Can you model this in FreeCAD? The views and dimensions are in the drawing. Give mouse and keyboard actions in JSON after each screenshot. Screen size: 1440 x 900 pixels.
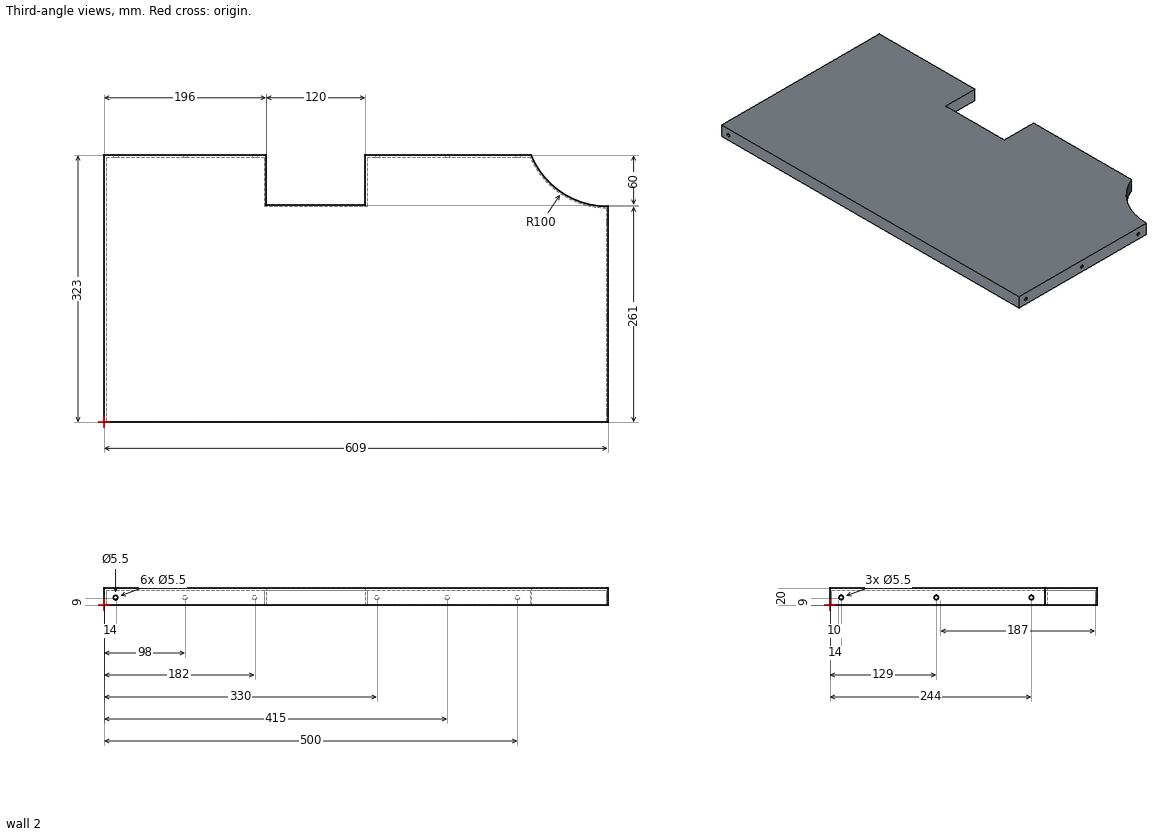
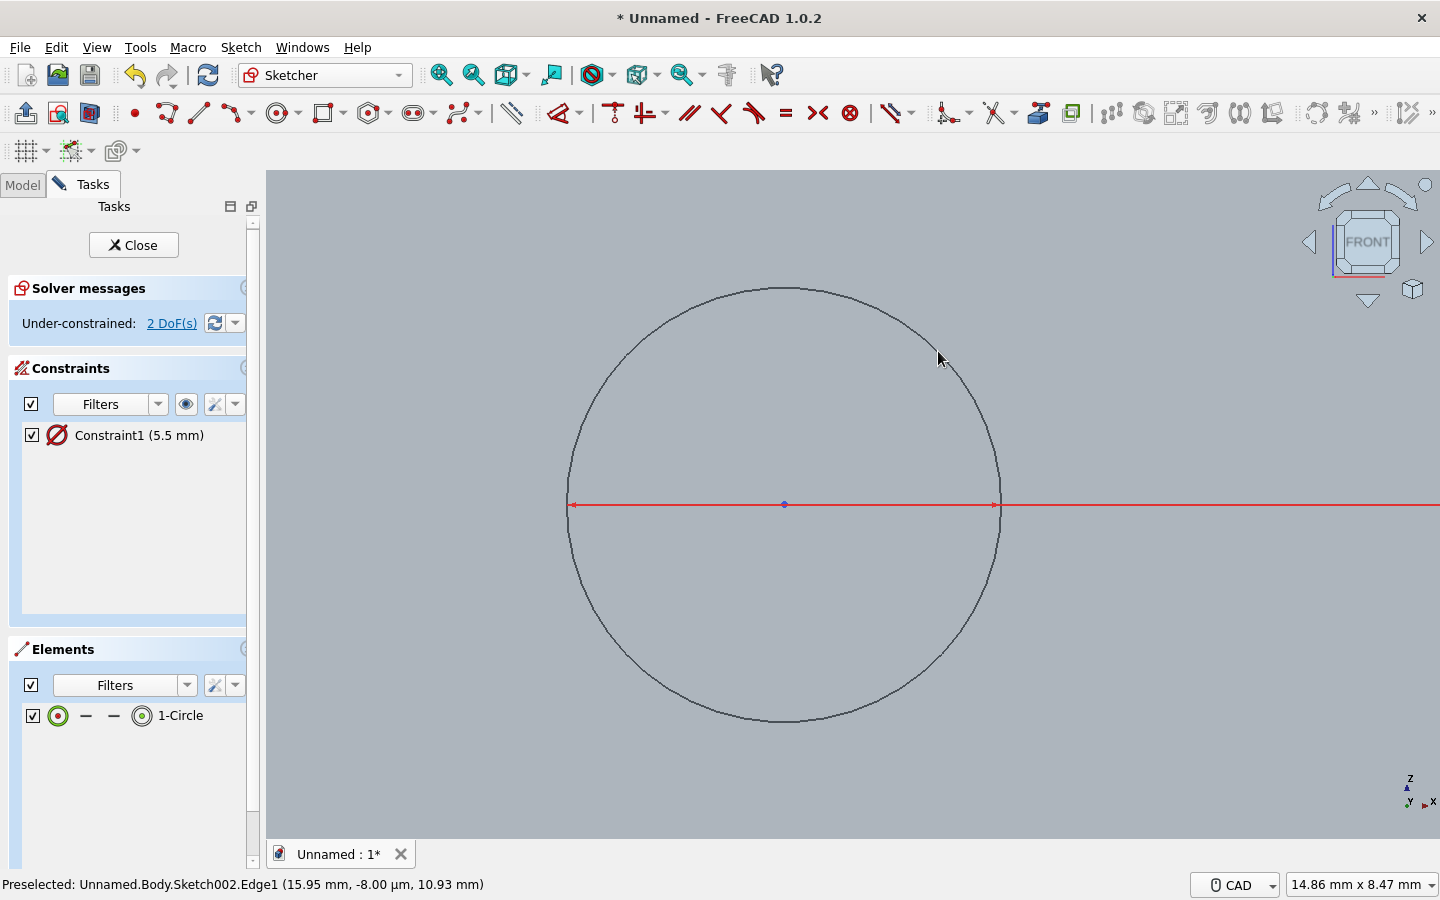
{"action": "key", "text": "d"}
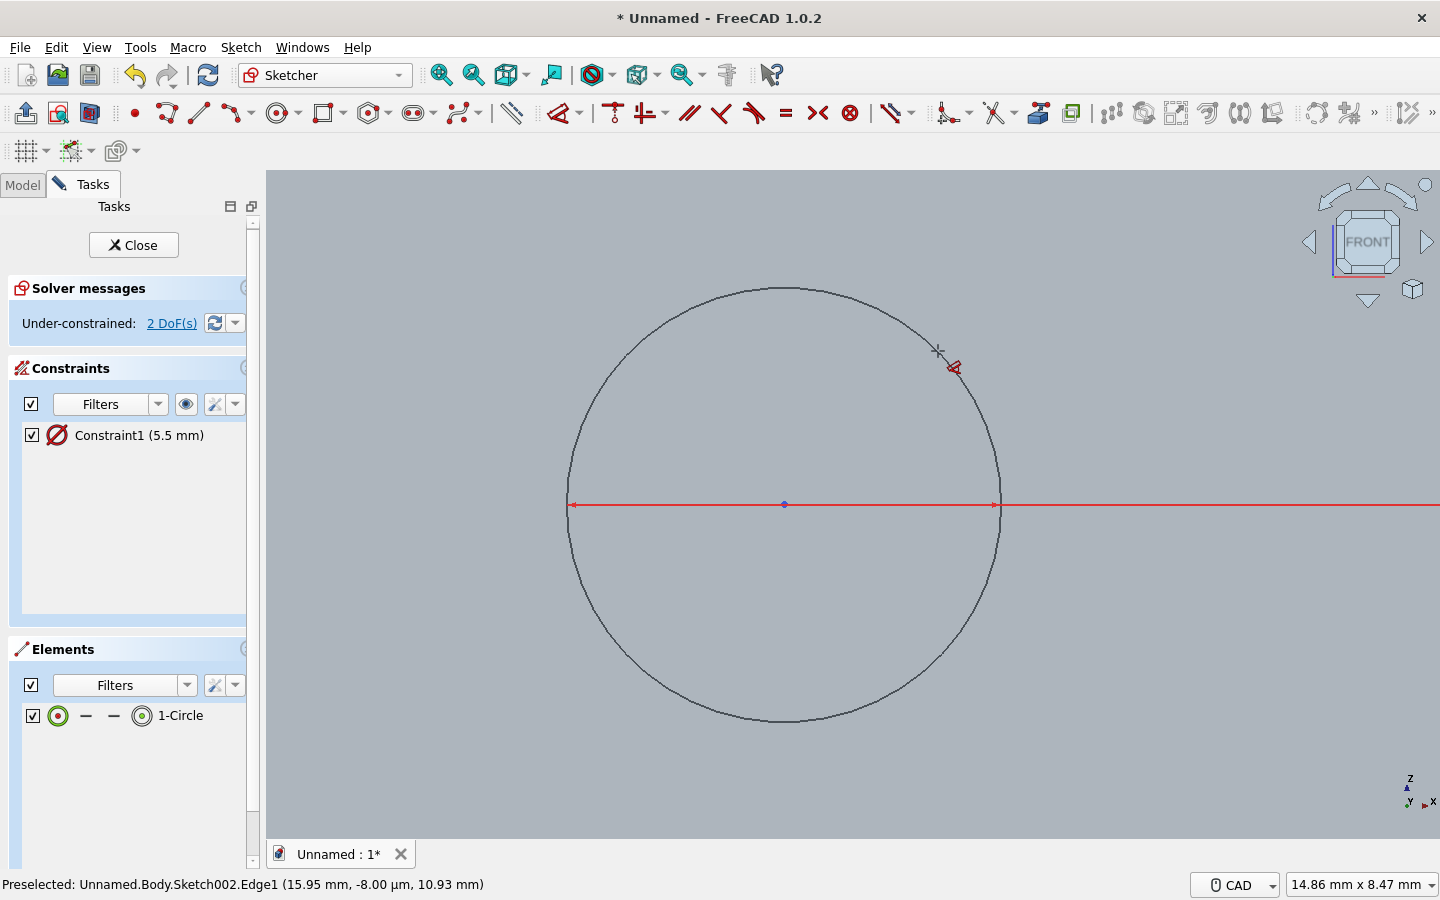
{"action": "left_click", "coordinate": [784, 505]}
{"action": "left_click", "coordinate": [818, 658]}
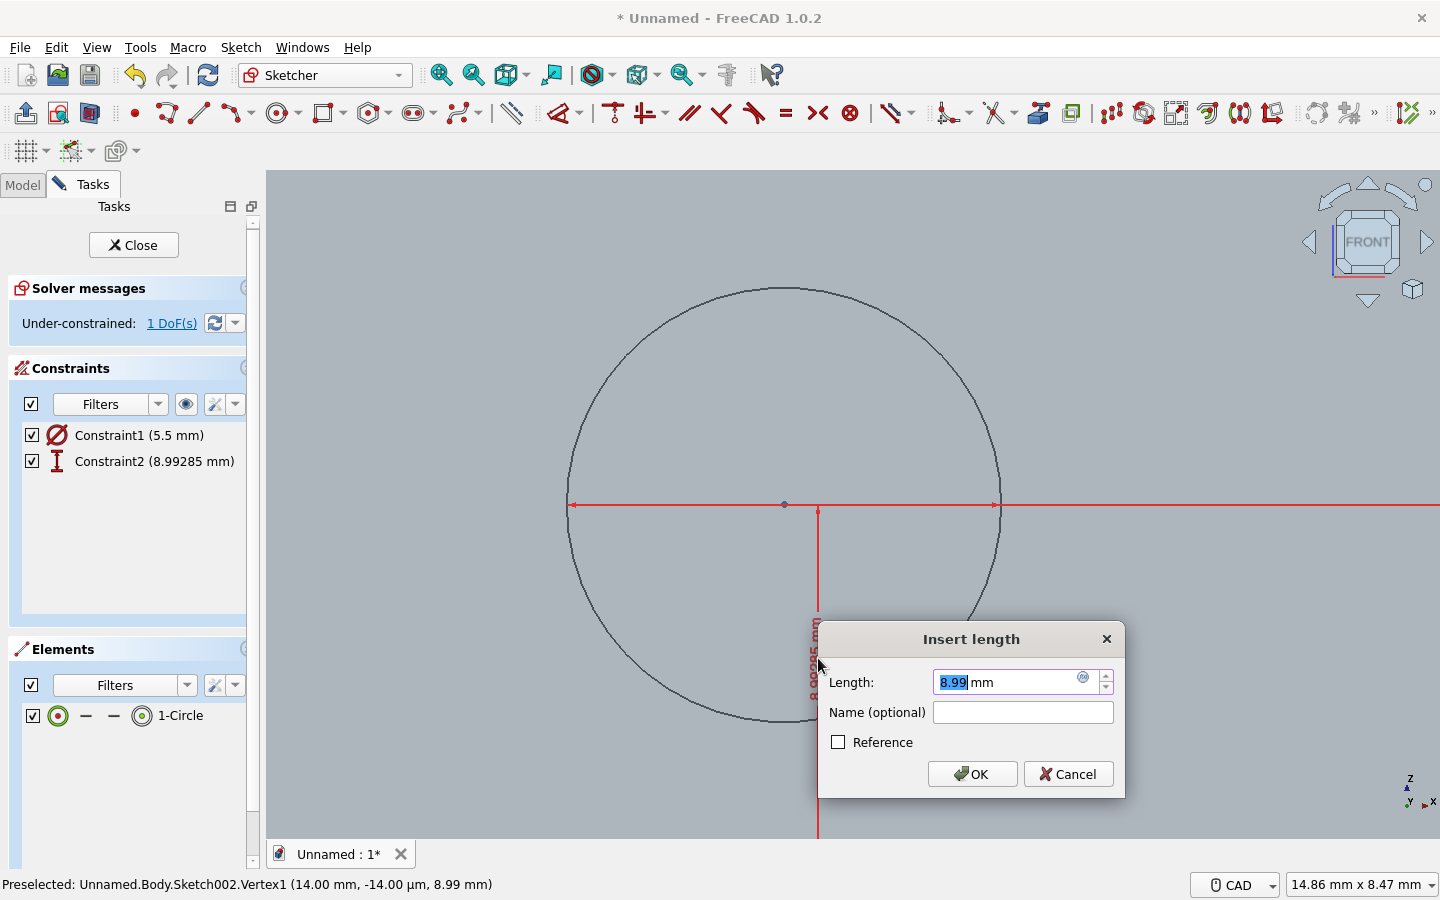
{"action": "type", "text": "9"}
{"action": "key", "text": "Return"}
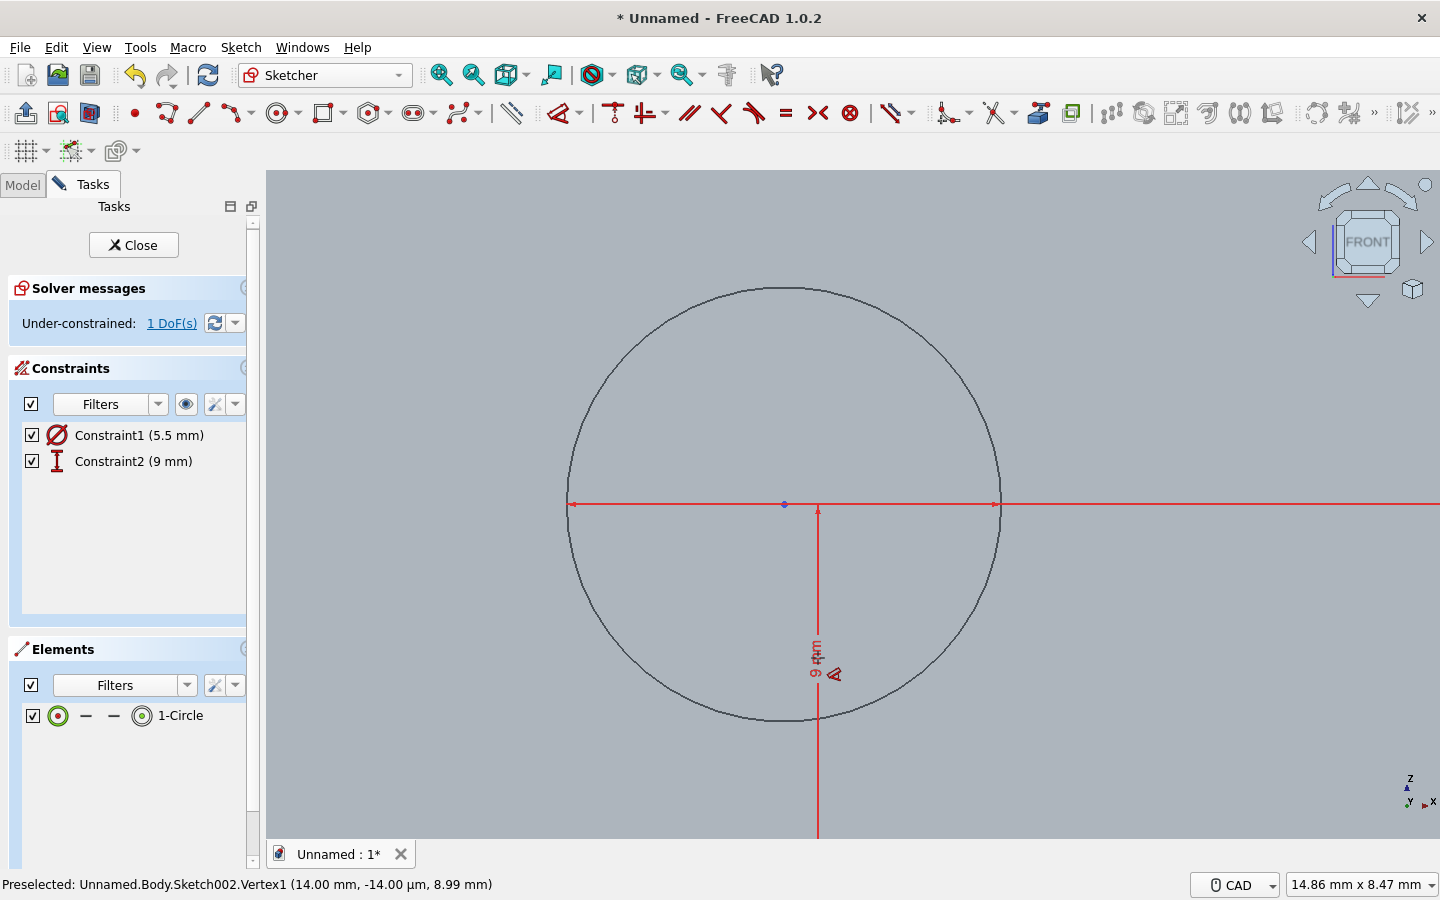
{"action": "left_click", "coordinate": [784, 504]}
{"action": "left_click", "coordinate": [539, 470]}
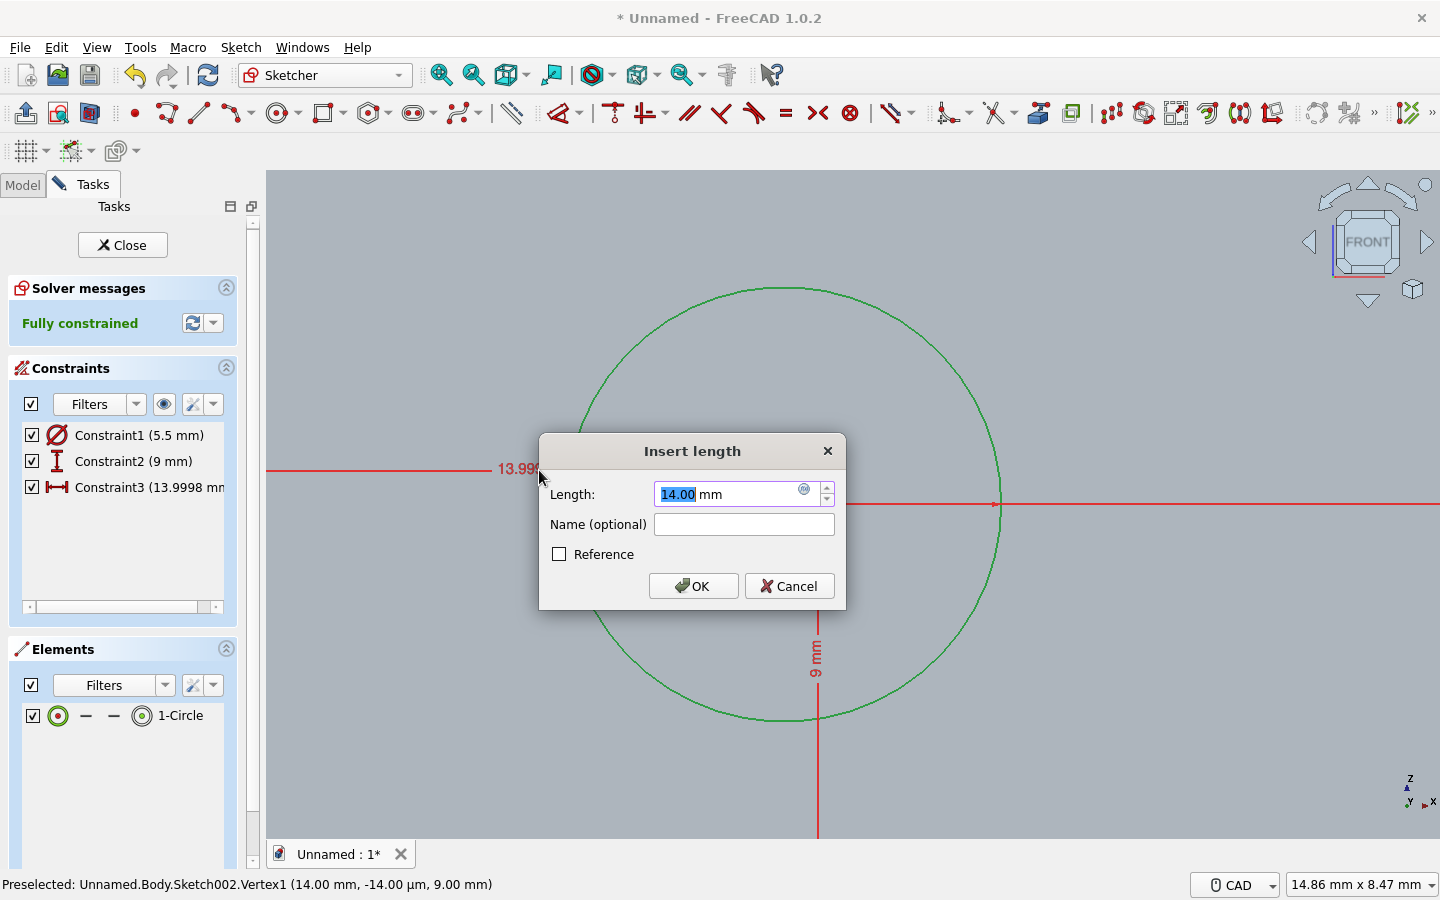
{"action": "type", "text": "14"}
{"action": "key", "text": "Return"}
{"action": "key", "text": "Escape"}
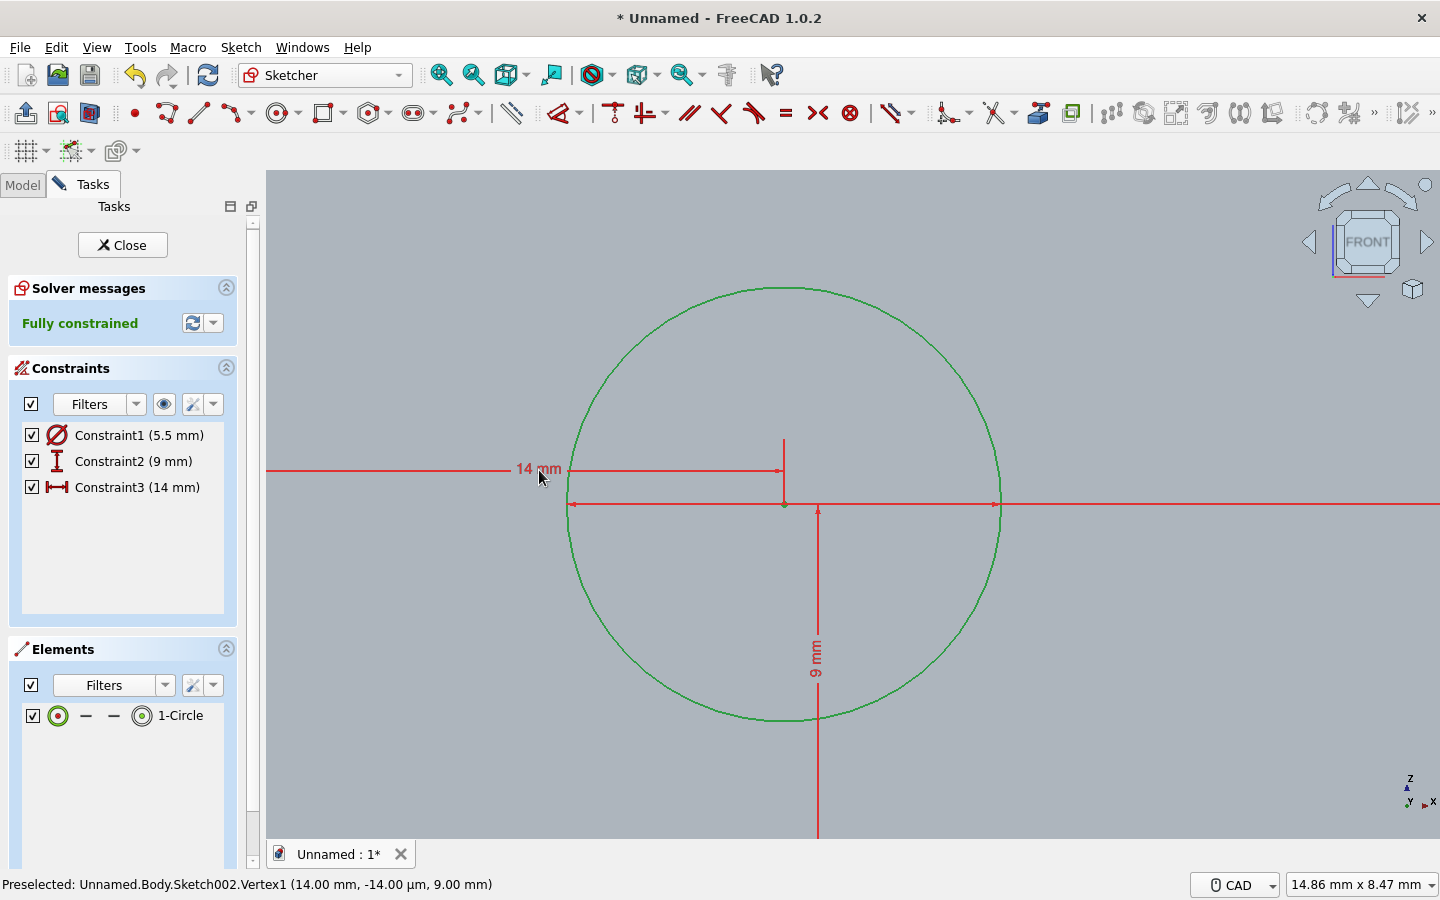
{"action": "left_click", "coordinate": [123, 245]}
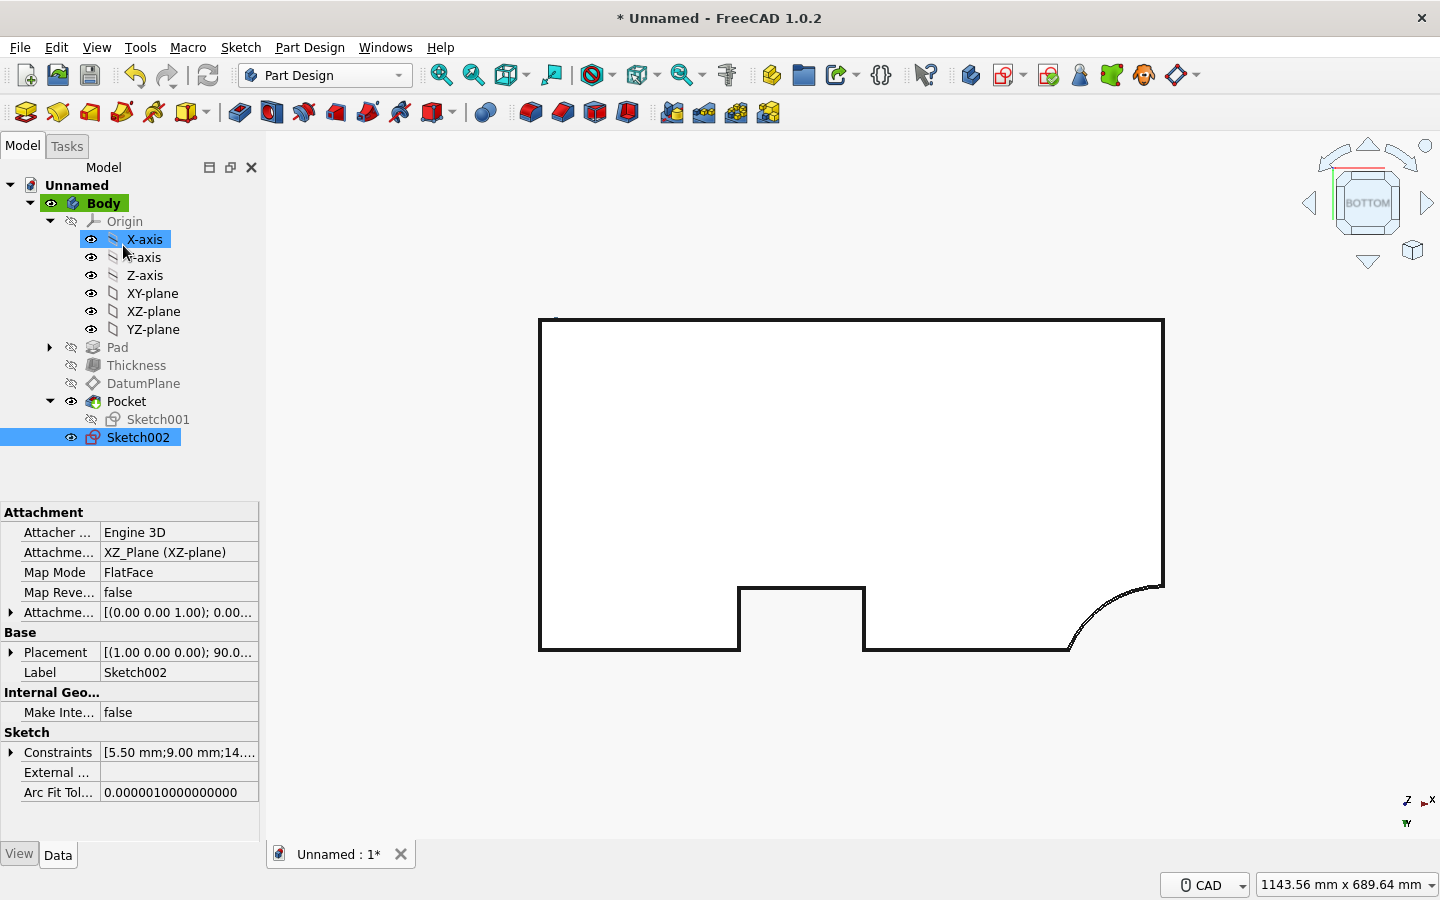
{"action": "left_click", "coordinate": [240, 112]}